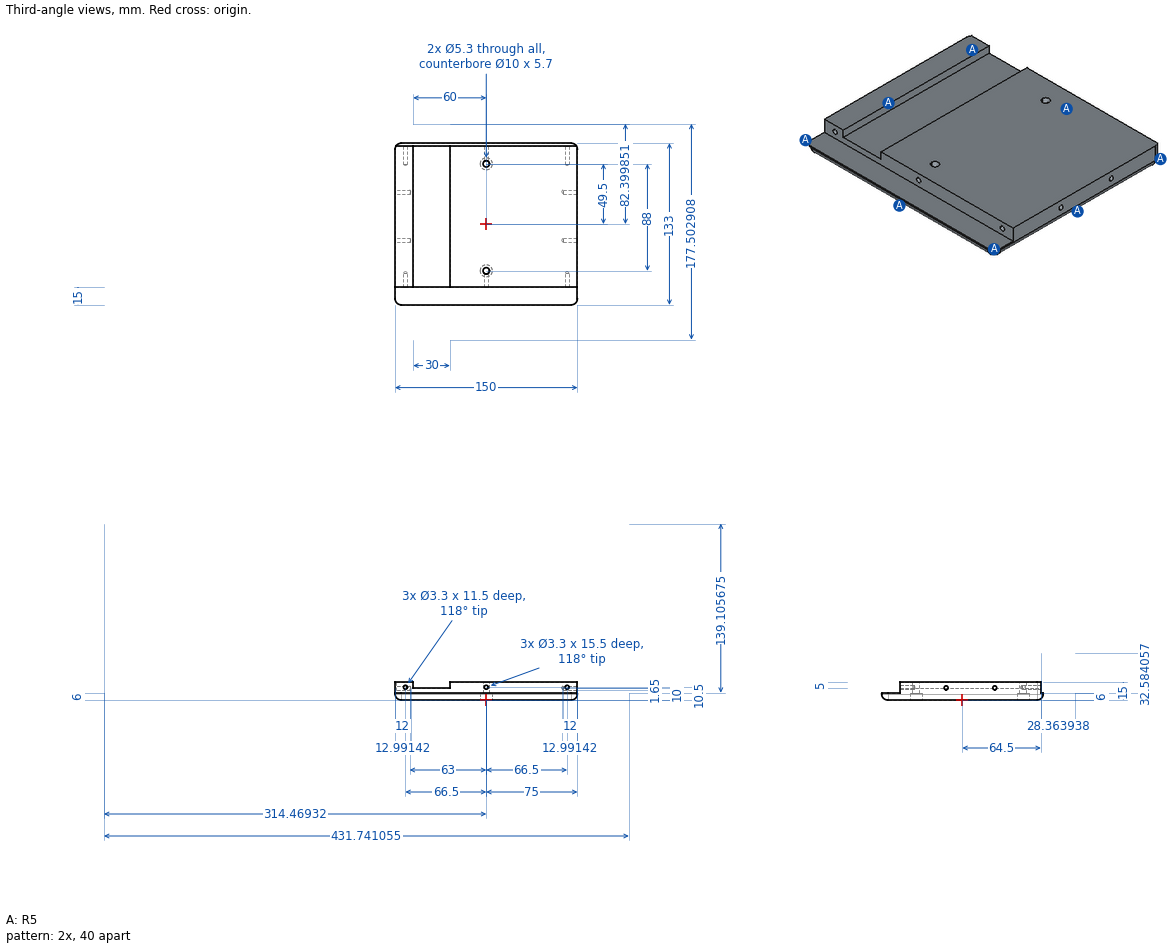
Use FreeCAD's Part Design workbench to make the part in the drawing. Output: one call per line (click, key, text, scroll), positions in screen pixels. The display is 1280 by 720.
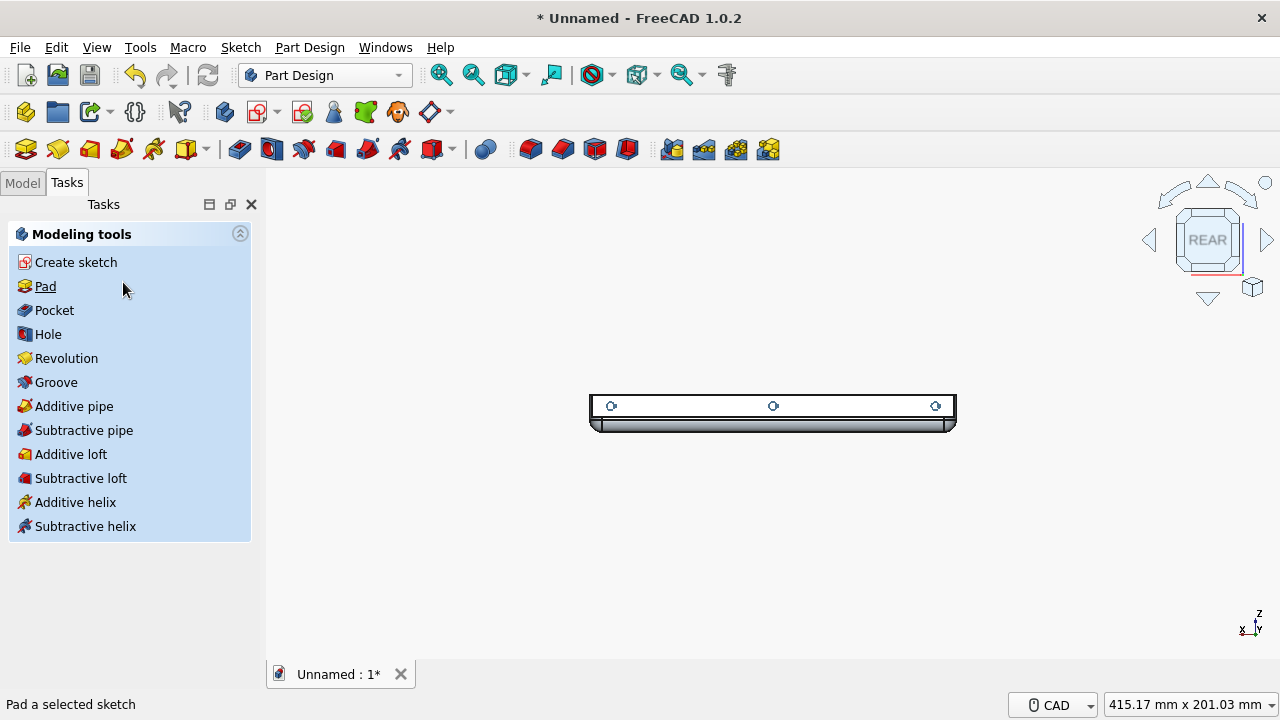
click(272, 150)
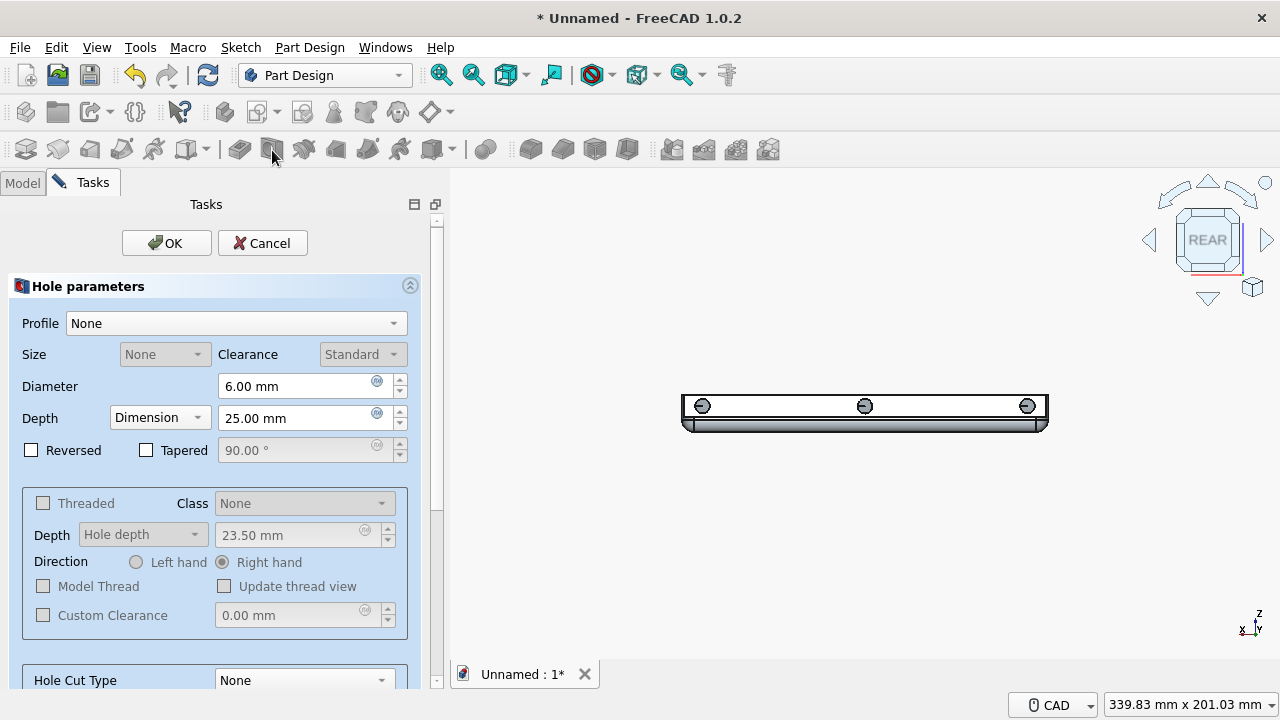
triple_click(305, 386)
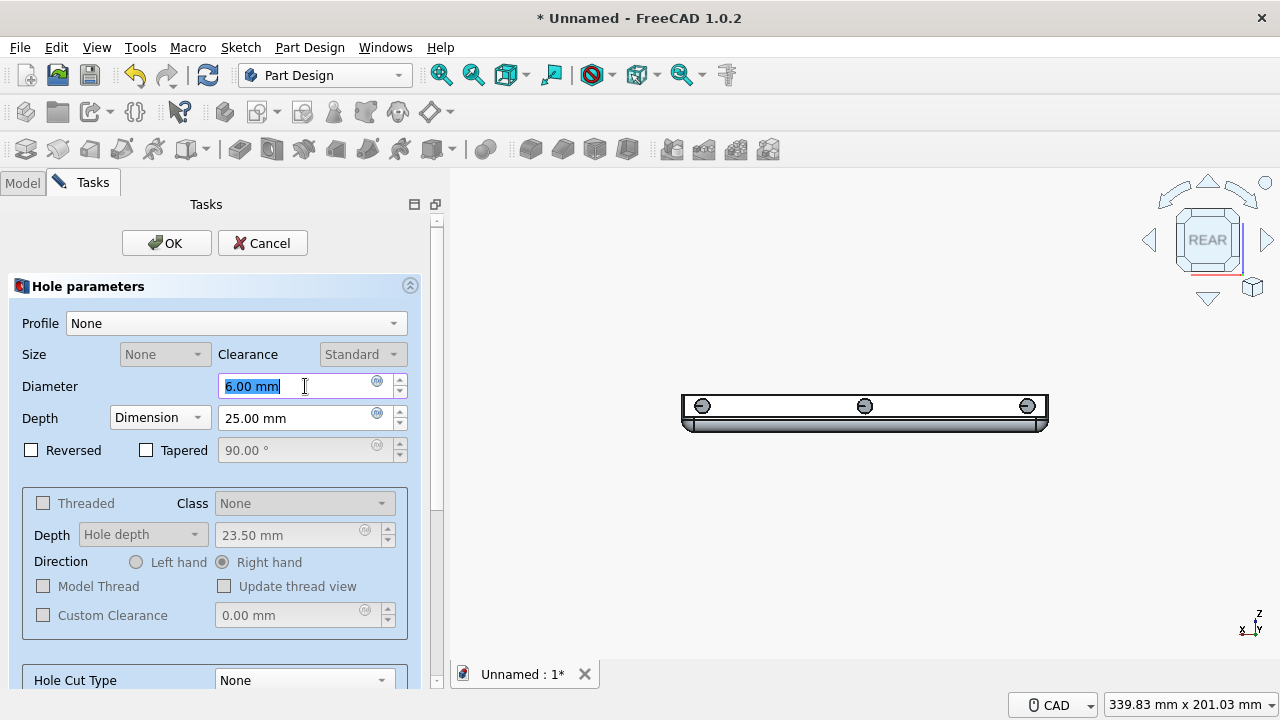
text(3.3)
key(Tab)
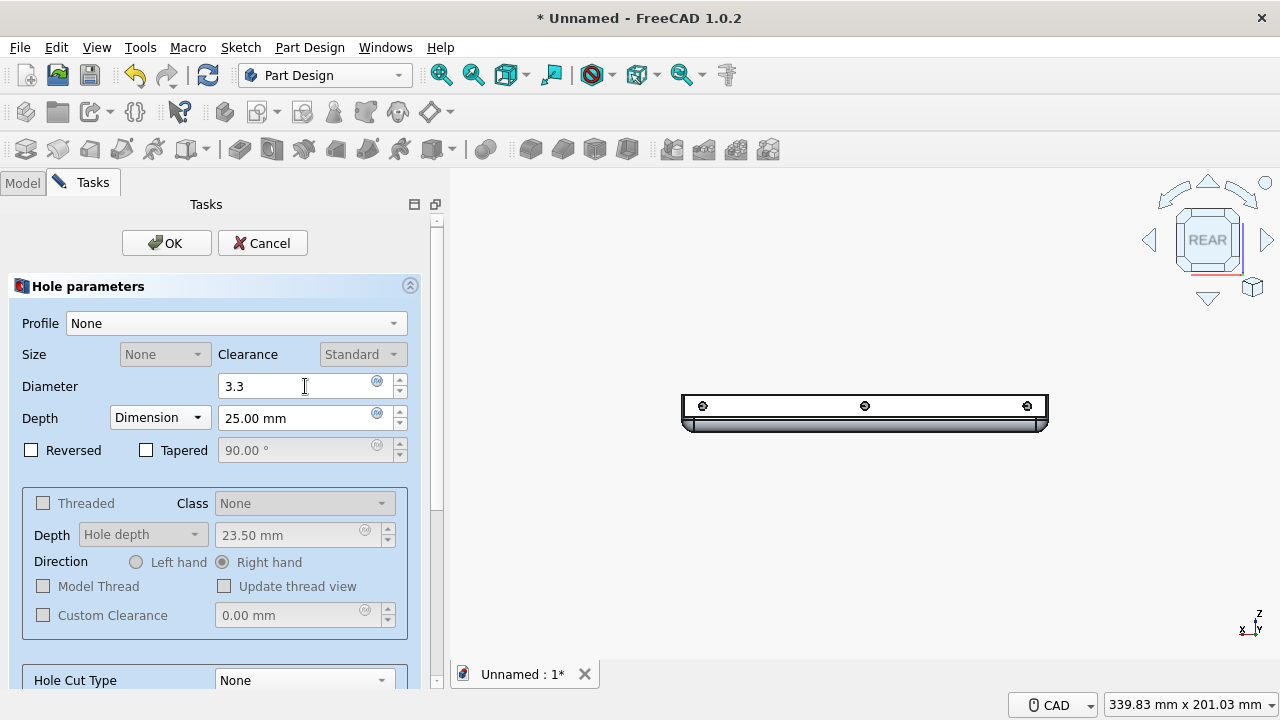
triple_click(305, 418)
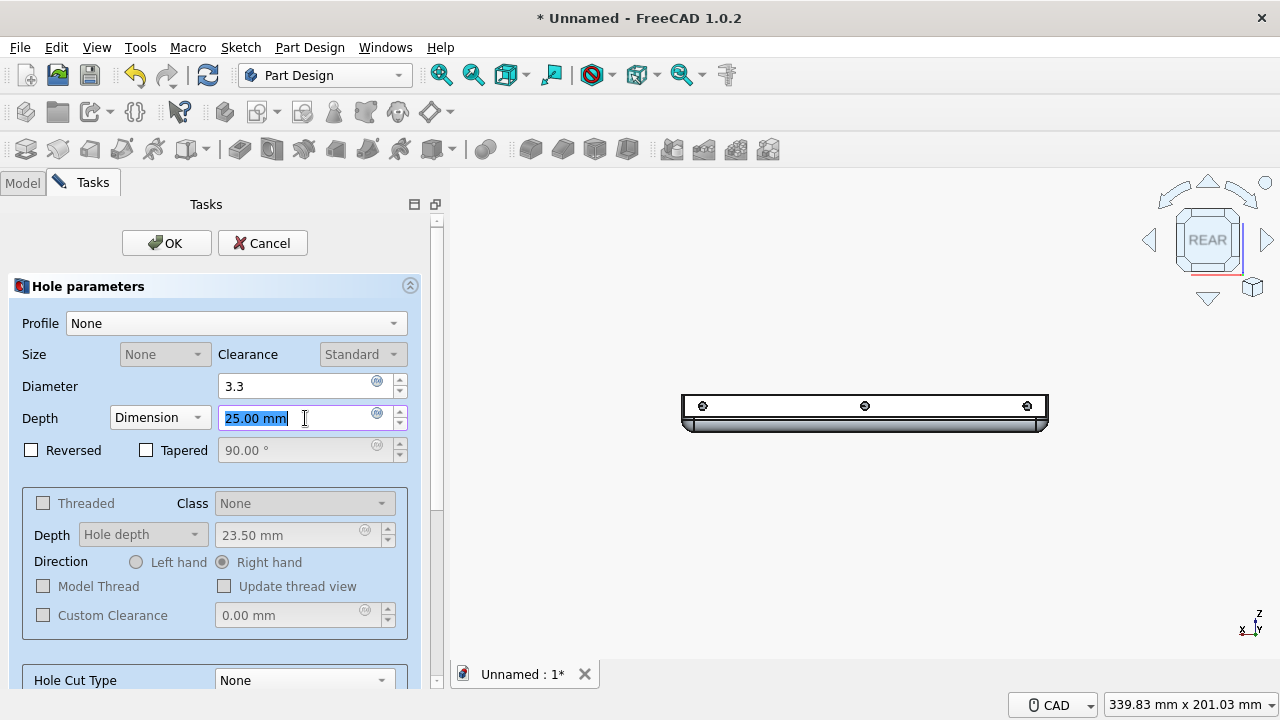
text(15.5)
key(Tab)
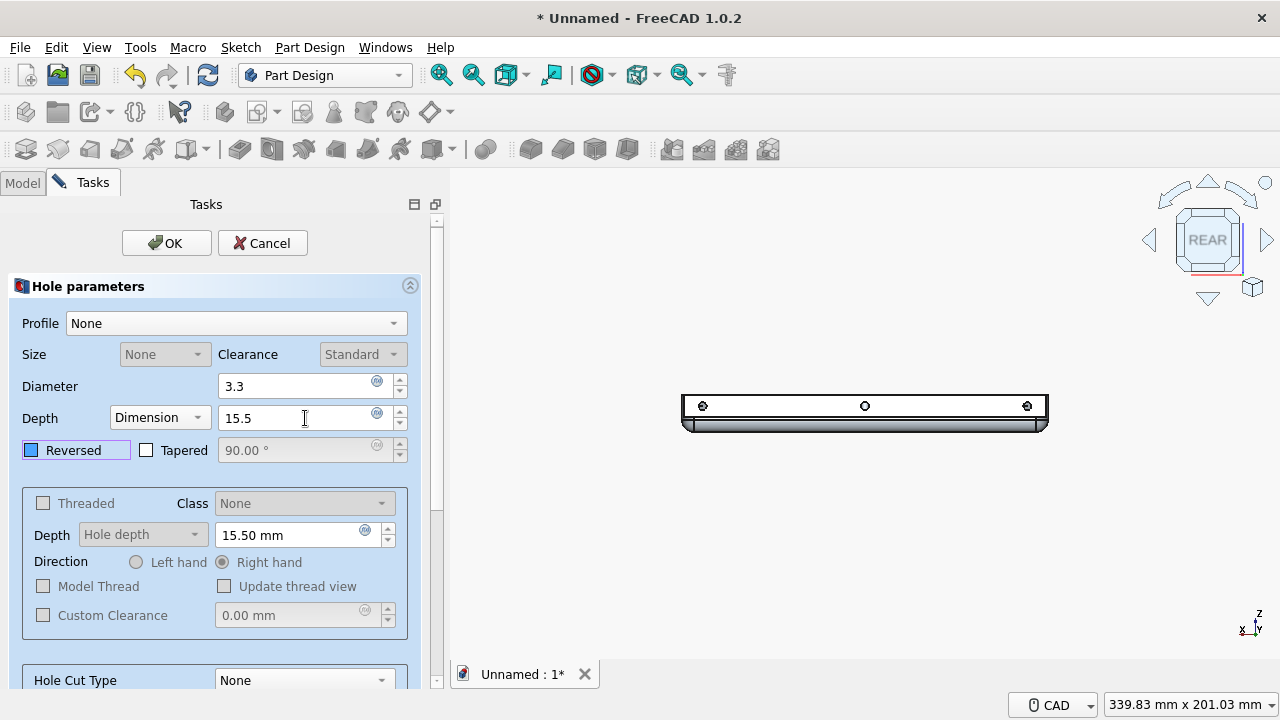
click(167, 243)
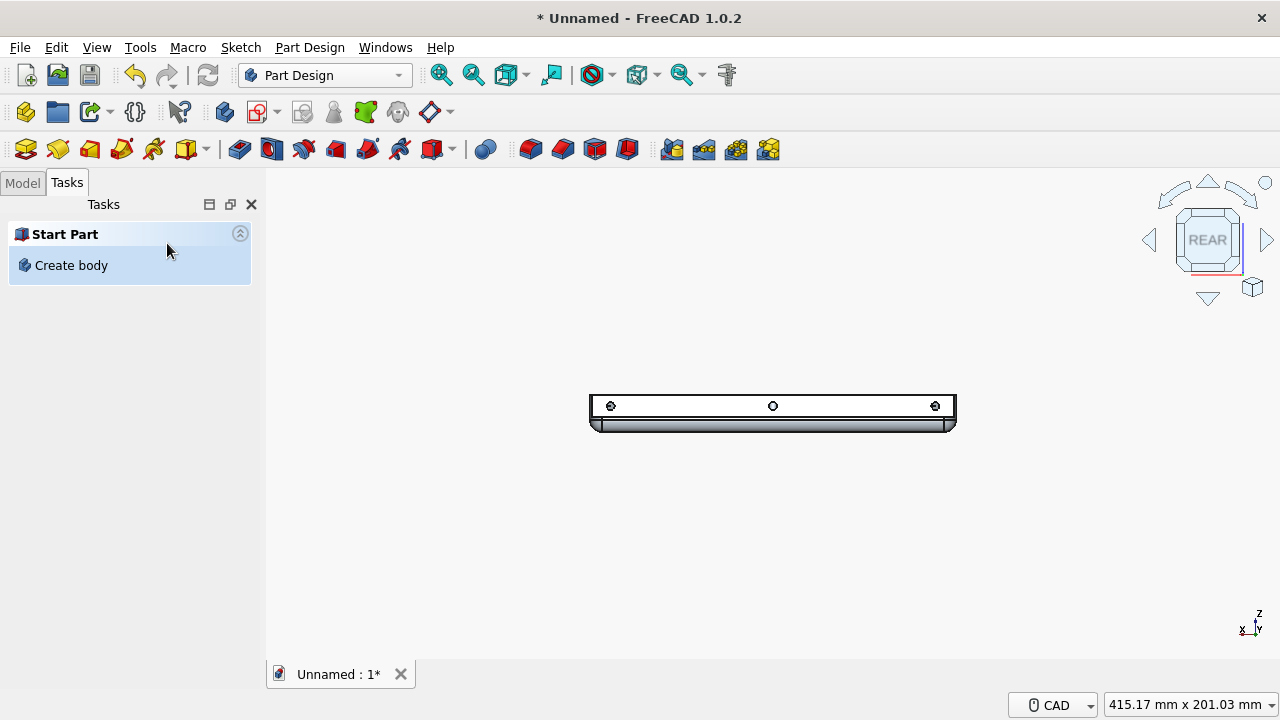
click(442, 76)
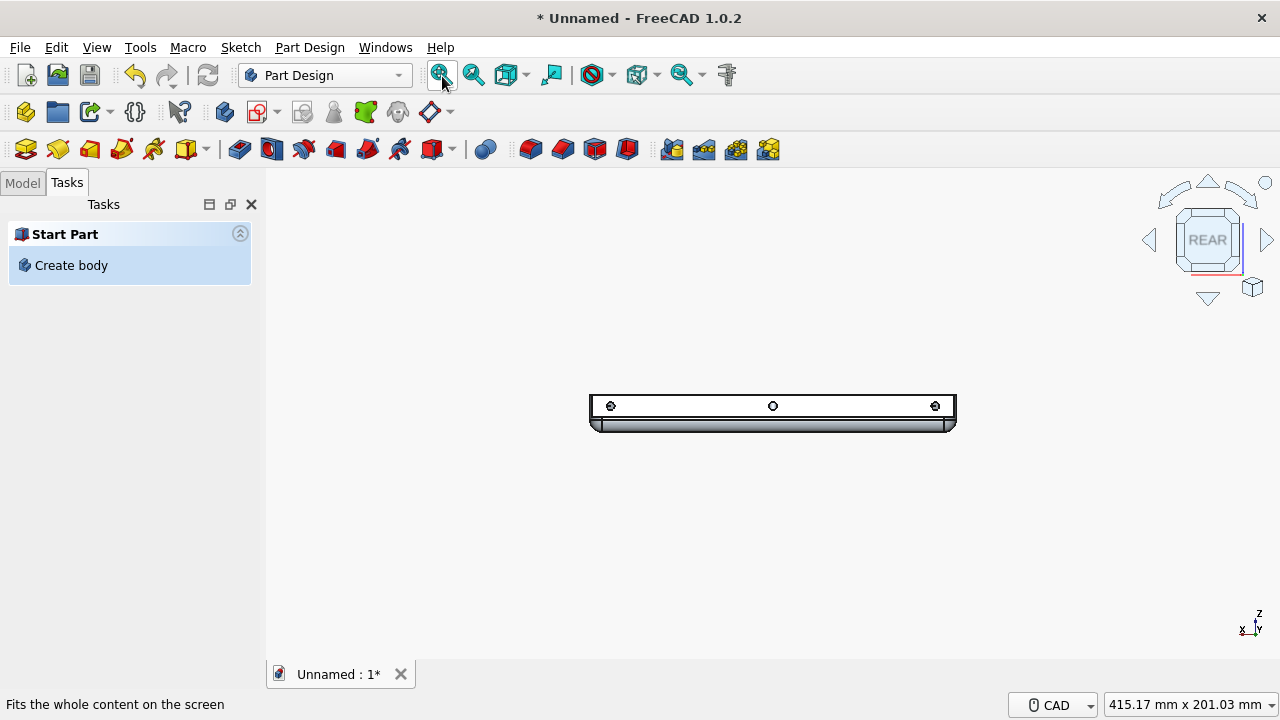
key(0)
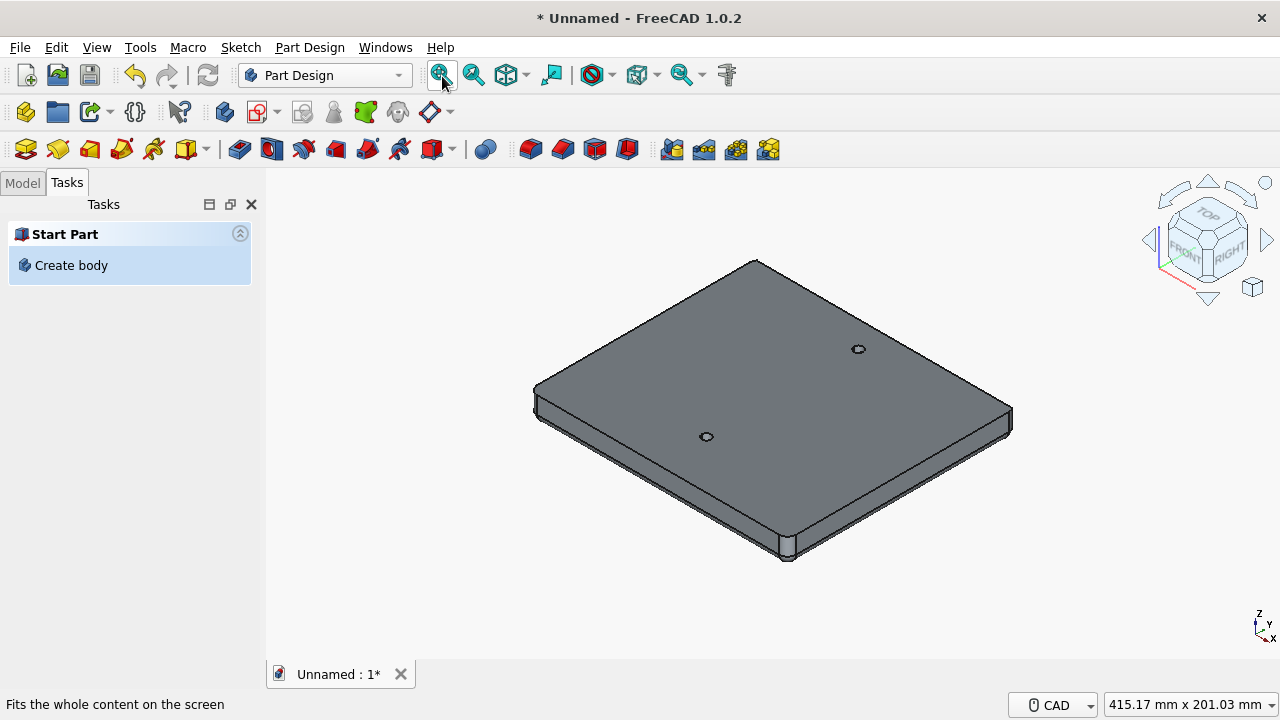
click(762, 536)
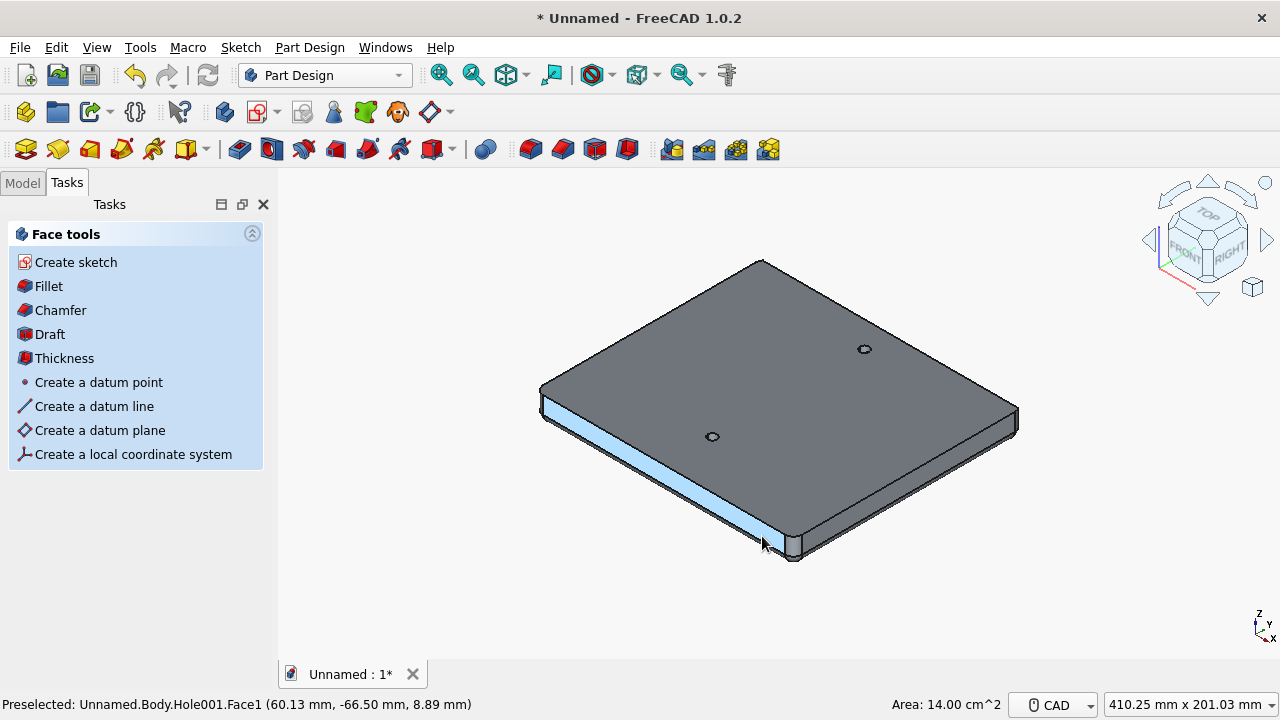
click(258, 112)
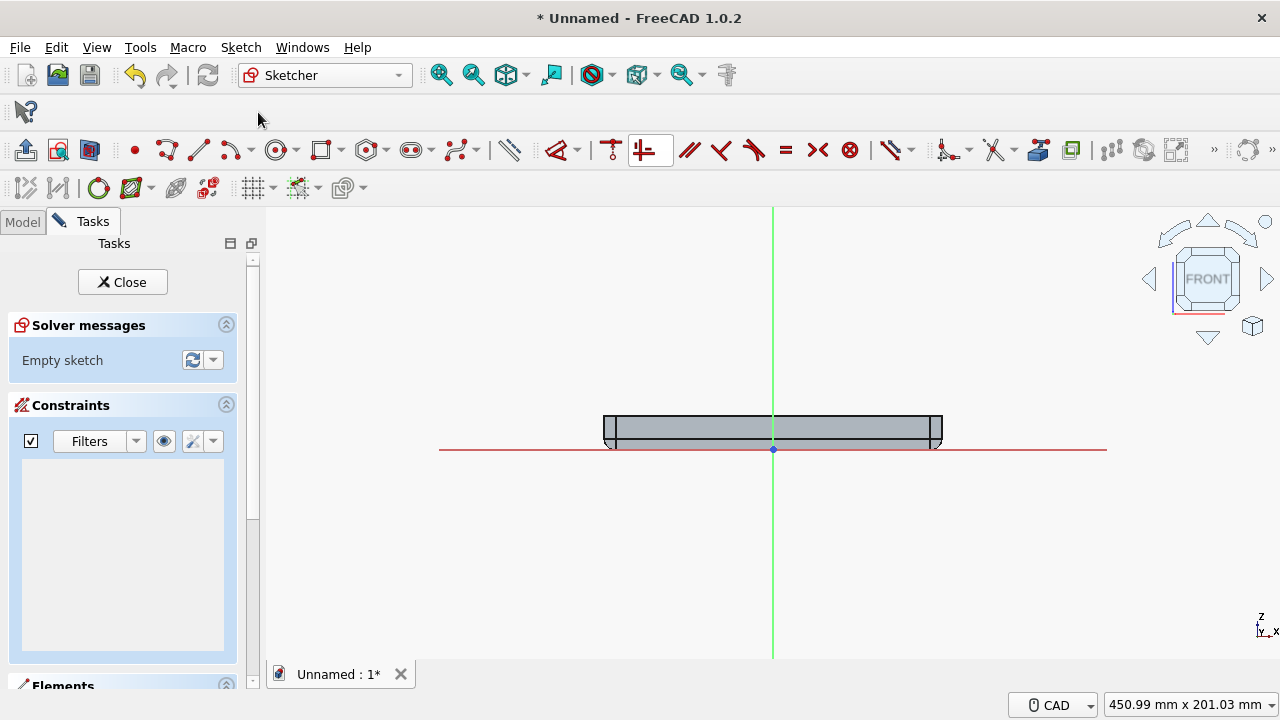
scroll(891, 611, down, 3)